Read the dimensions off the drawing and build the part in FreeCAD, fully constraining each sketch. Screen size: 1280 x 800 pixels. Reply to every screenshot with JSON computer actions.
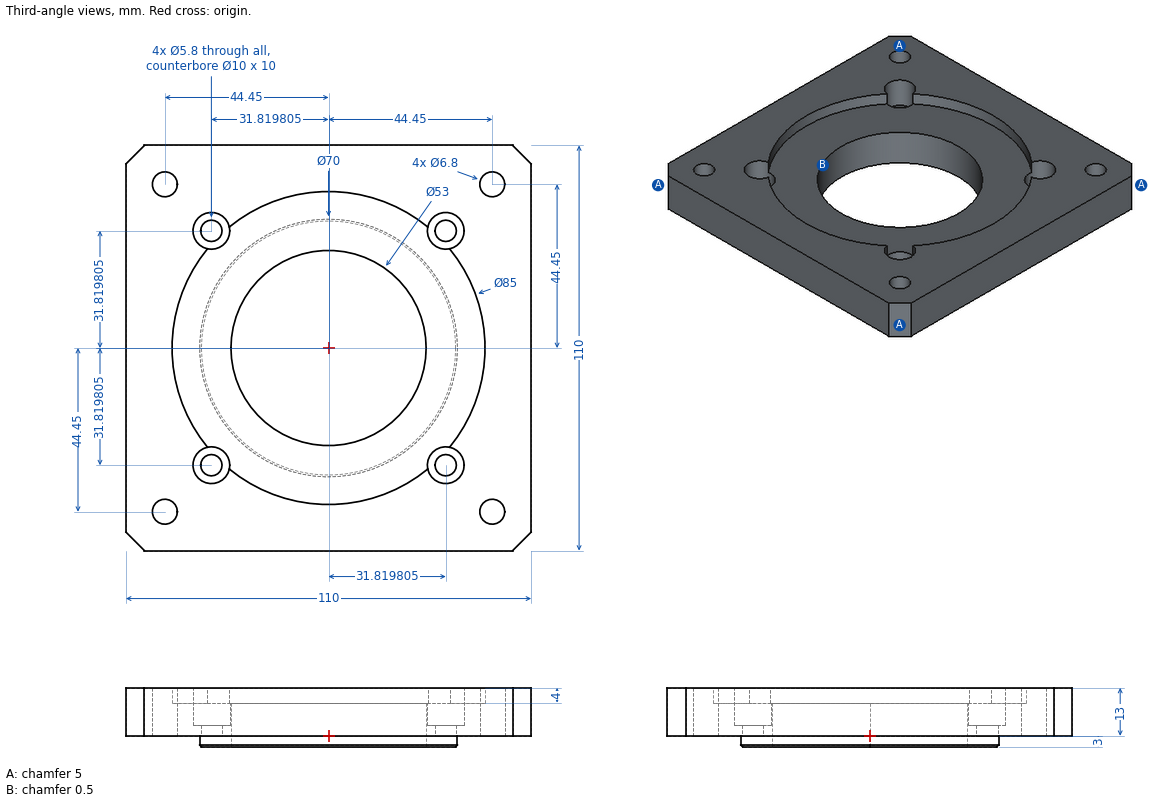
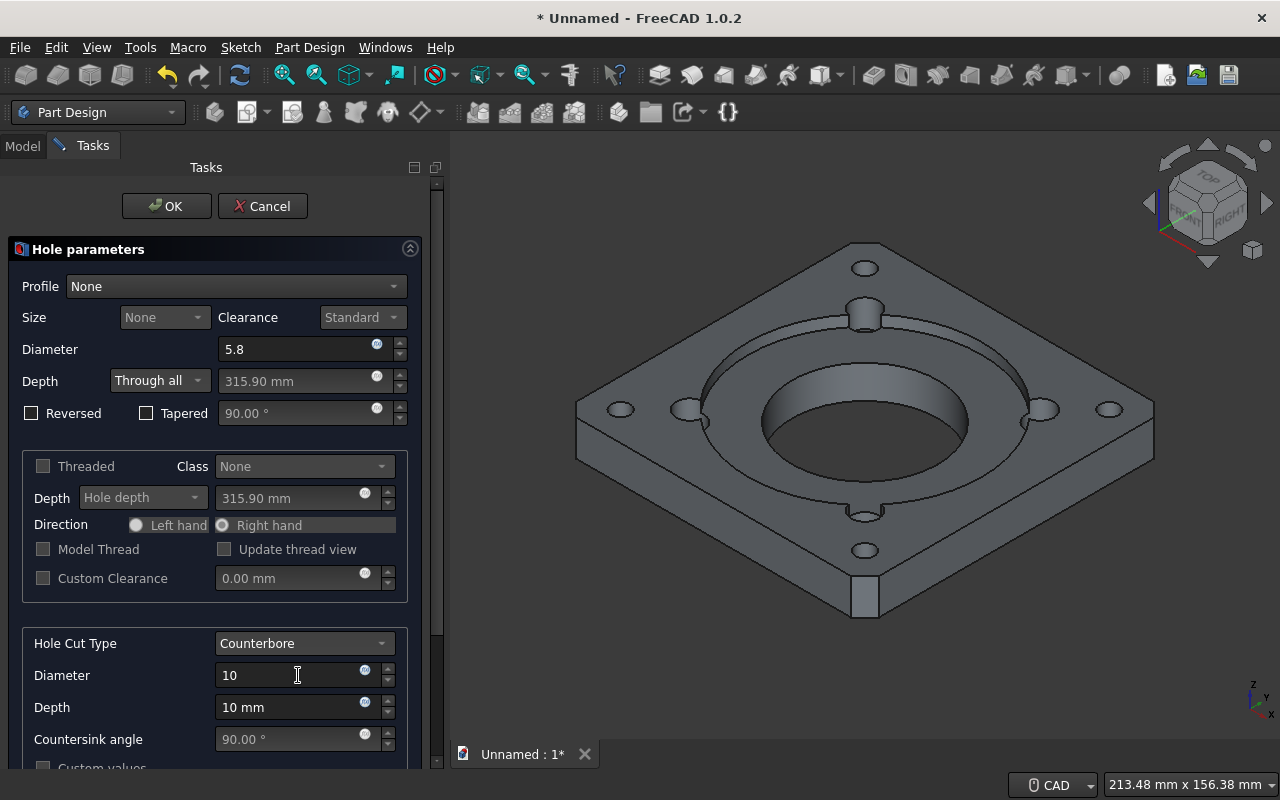
{"action": "left_click", "coordinate": [167, 206]}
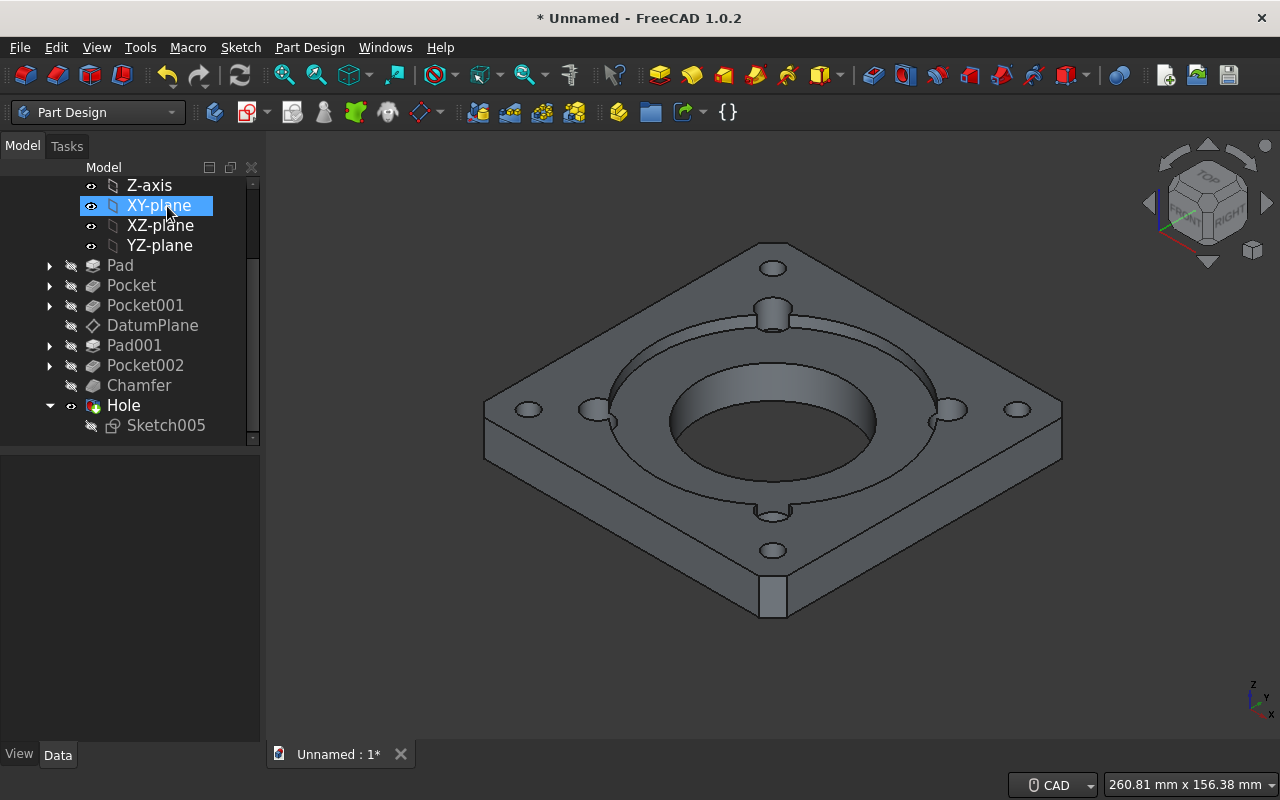
{"action": "key", "text": "2"}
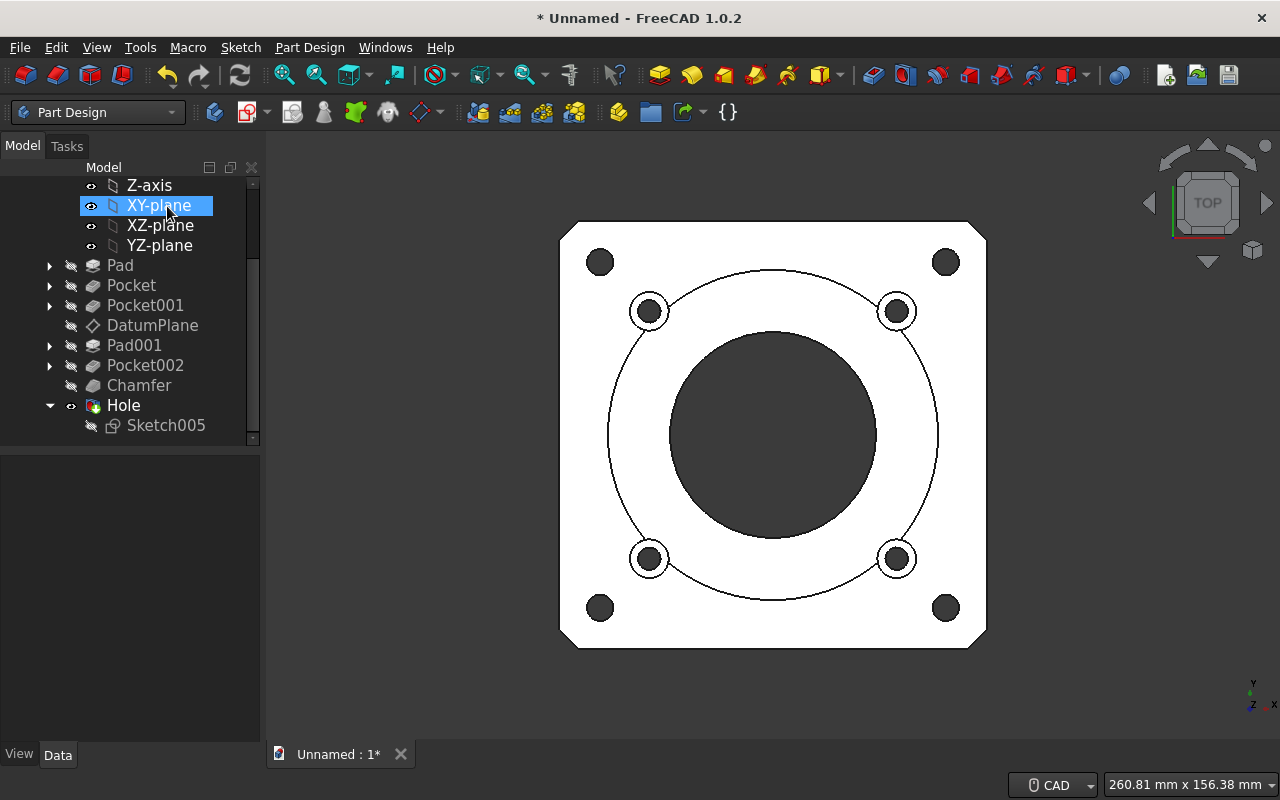
{"action": "key", "text": "0"}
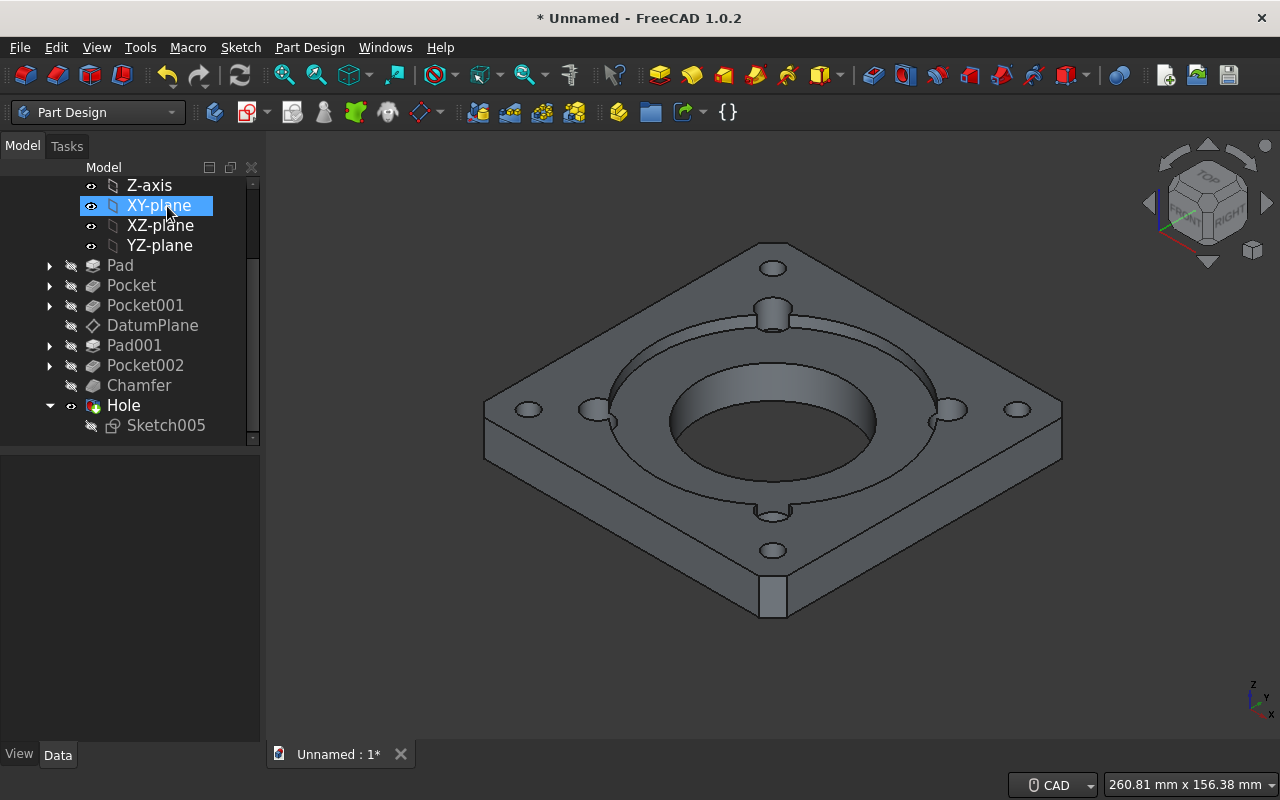
{"action": "key", "text": "1"}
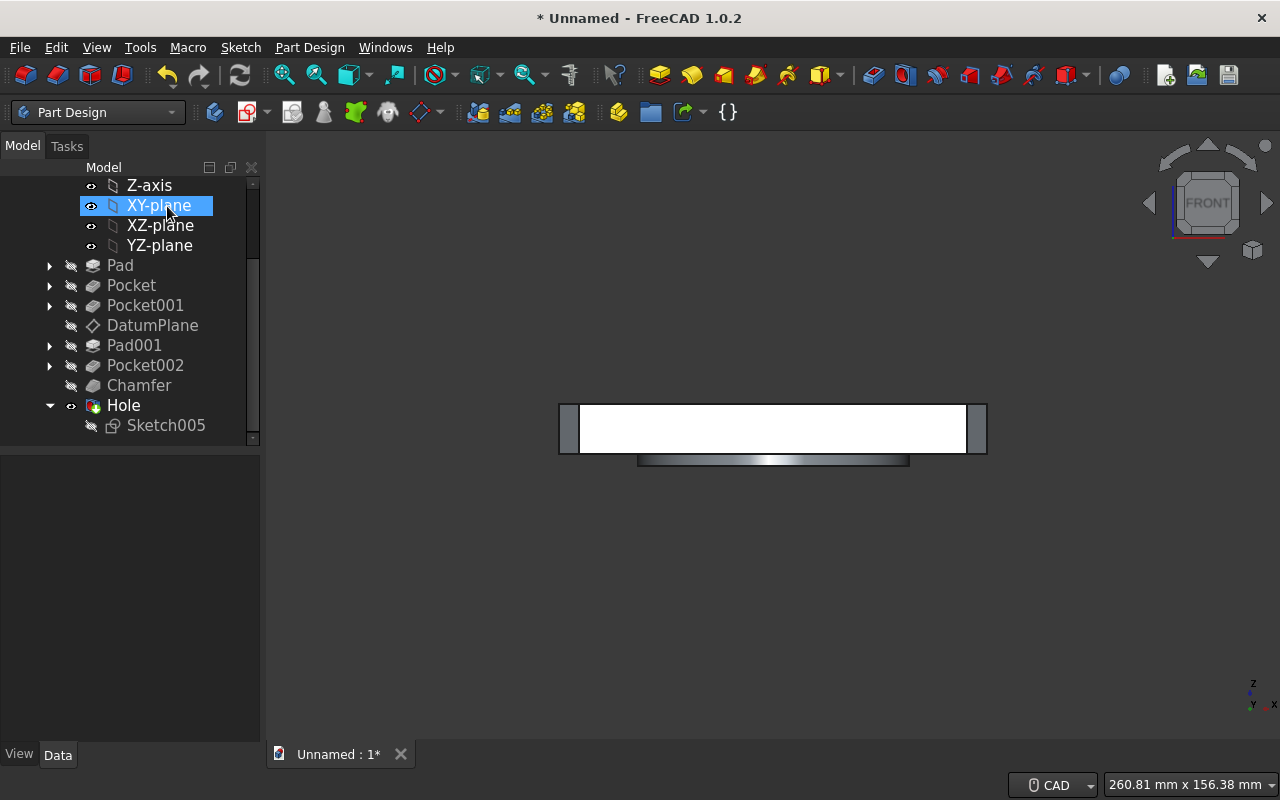
{"action": "left_click", "coordinate": [286, 76]}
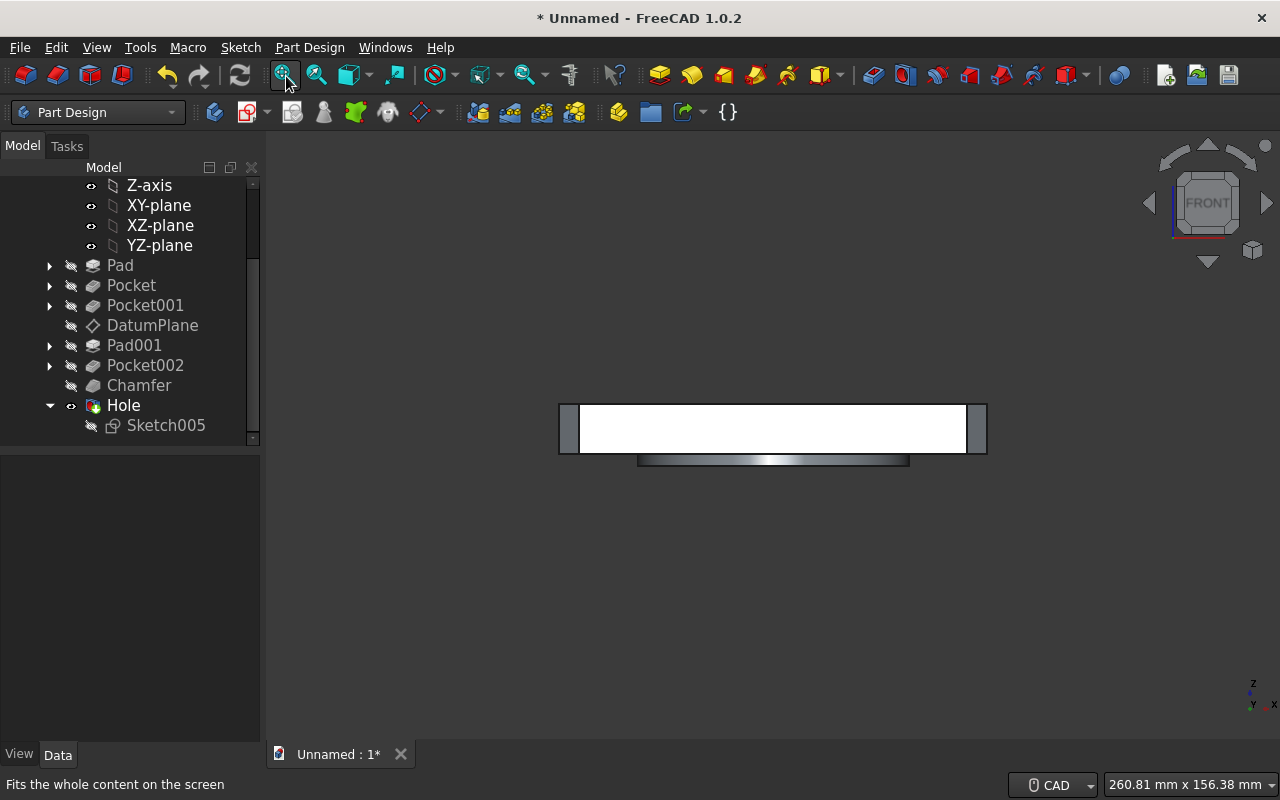
{"action": "left_click", "coordinate": [663, 465]}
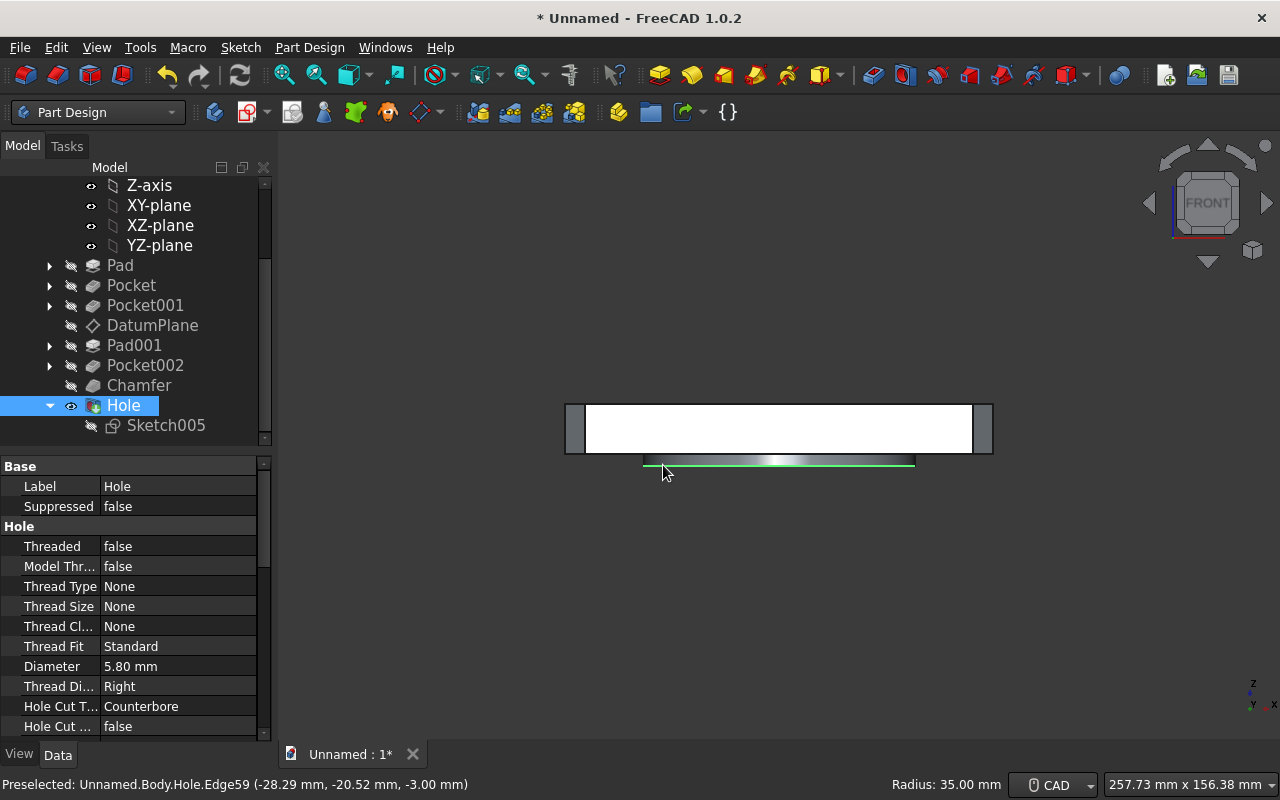
{"action": "left_click", "coordinate": [58, 76]}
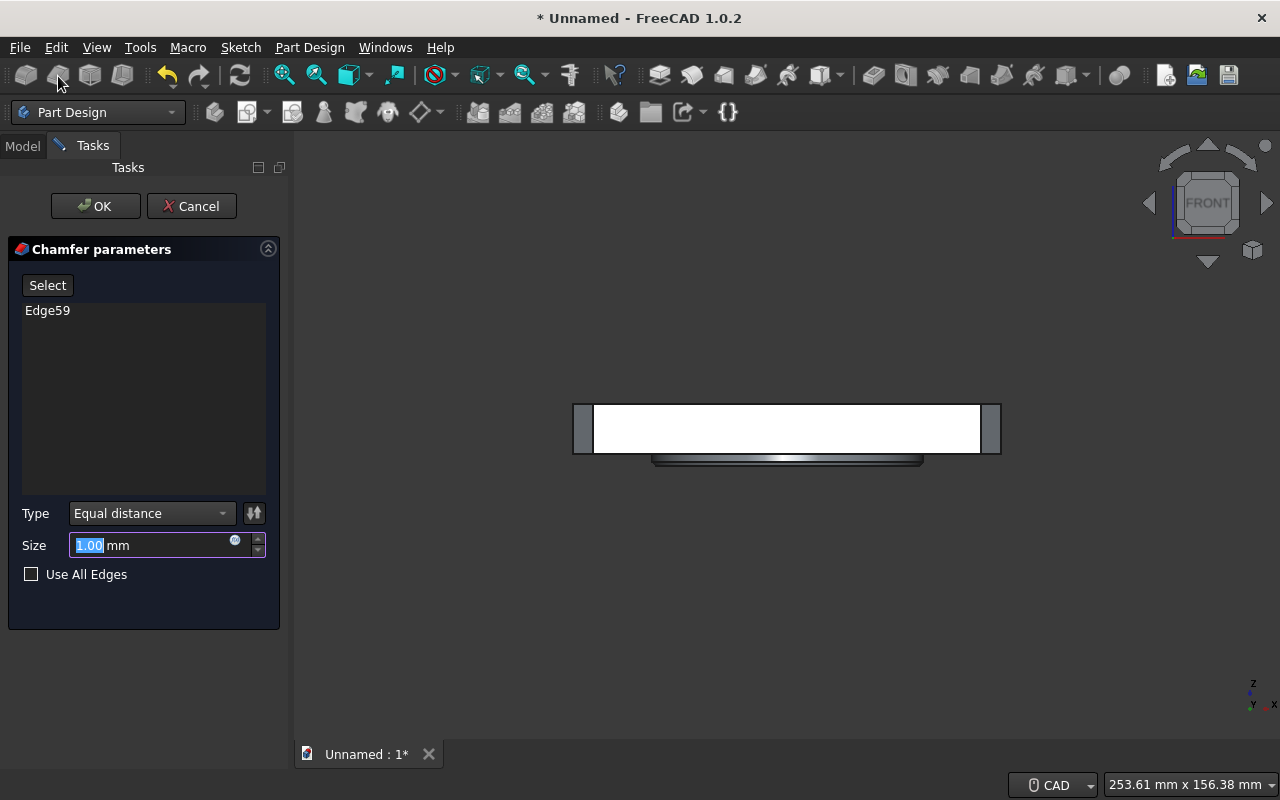
{"action": "type", "text": "0.5"}
{"action": "key", "text": "Tab"}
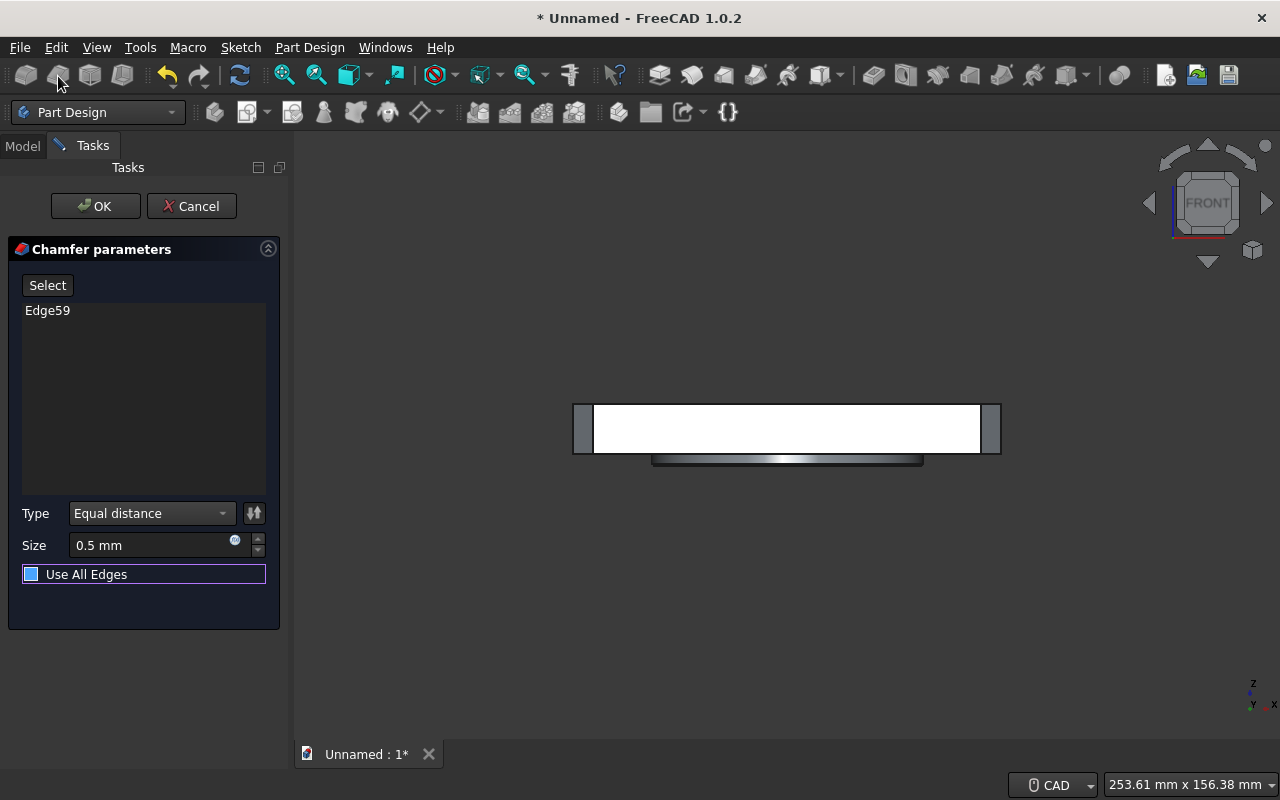
{"action": "left_click", "coordinate": [96, 206]}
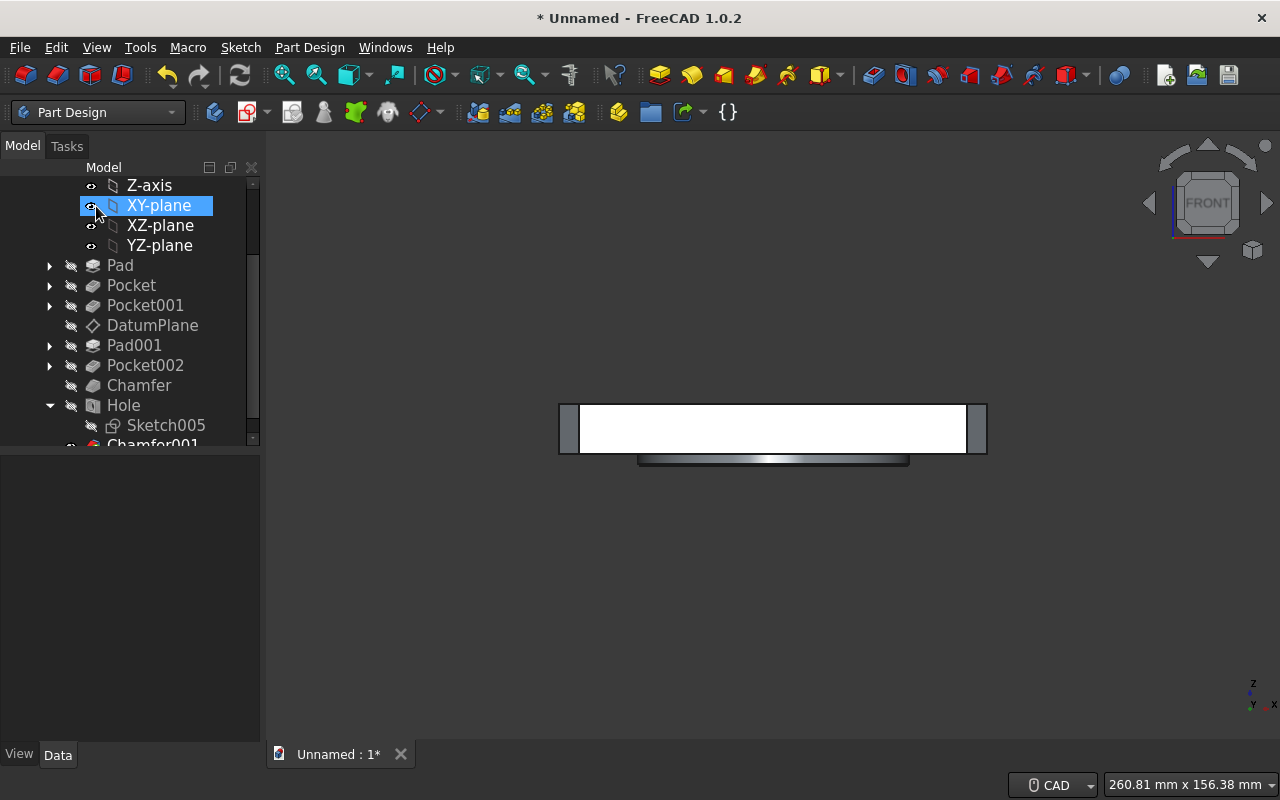
{"action": "key", "text": "0"}